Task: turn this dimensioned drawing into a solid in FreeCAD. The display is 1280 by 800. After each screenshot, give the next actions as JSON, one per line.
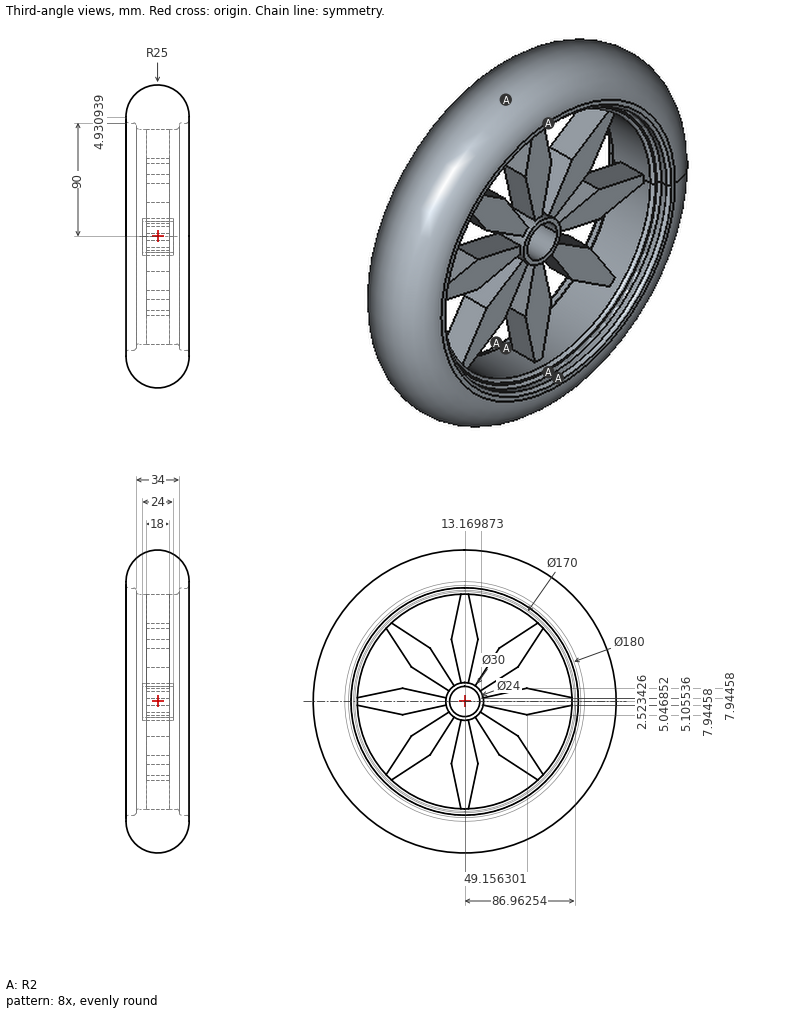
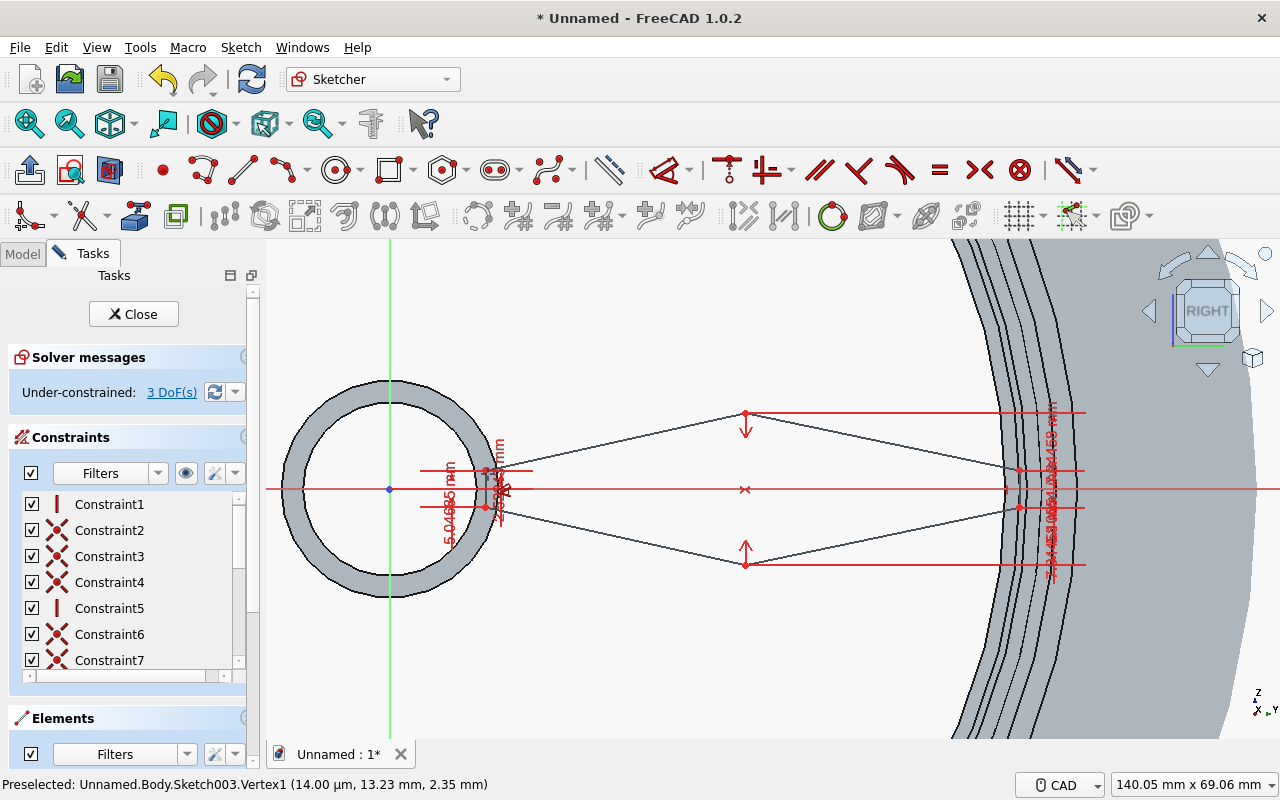
{"action": "left_click", "coordinate": [1020, 508]}
{"action": "left_click", "coordinate": [705, 542]}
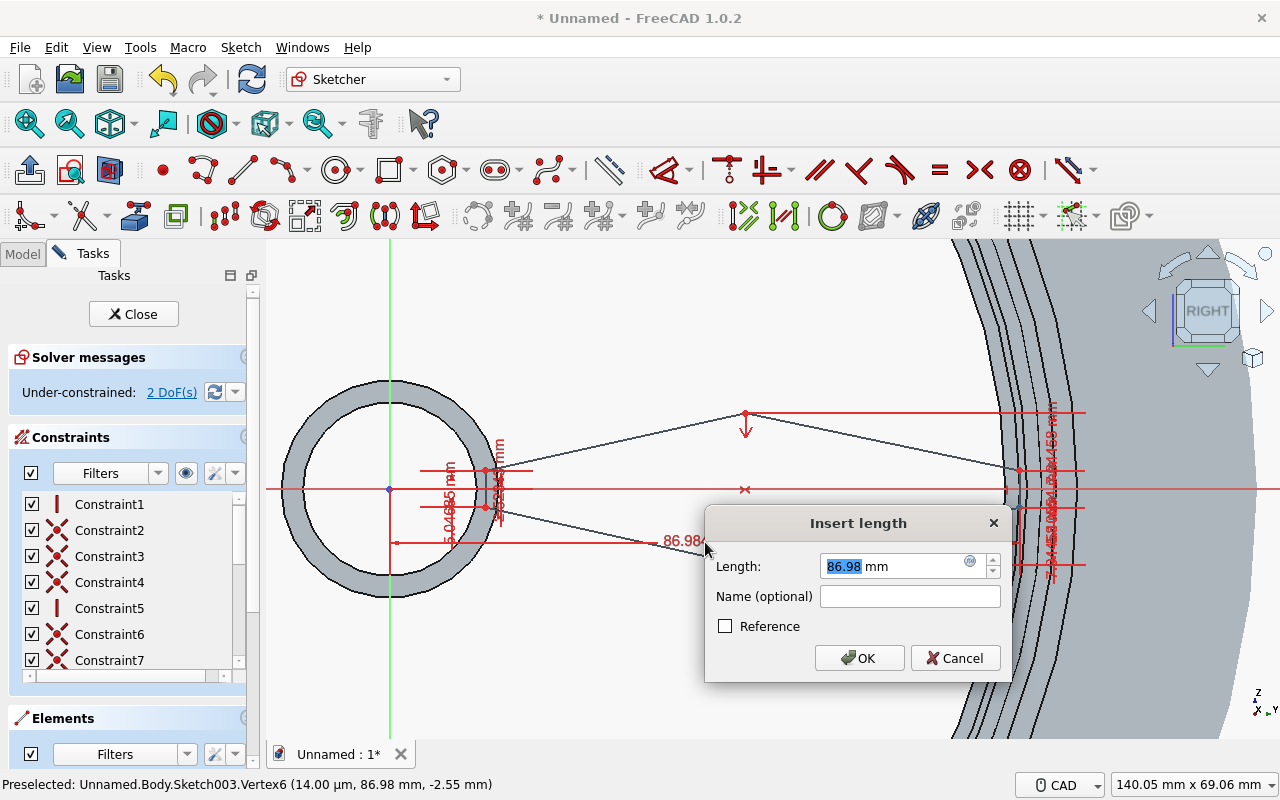
{"action": "type", "text": "86.96254"}
{"action": "key", "text": "Return"}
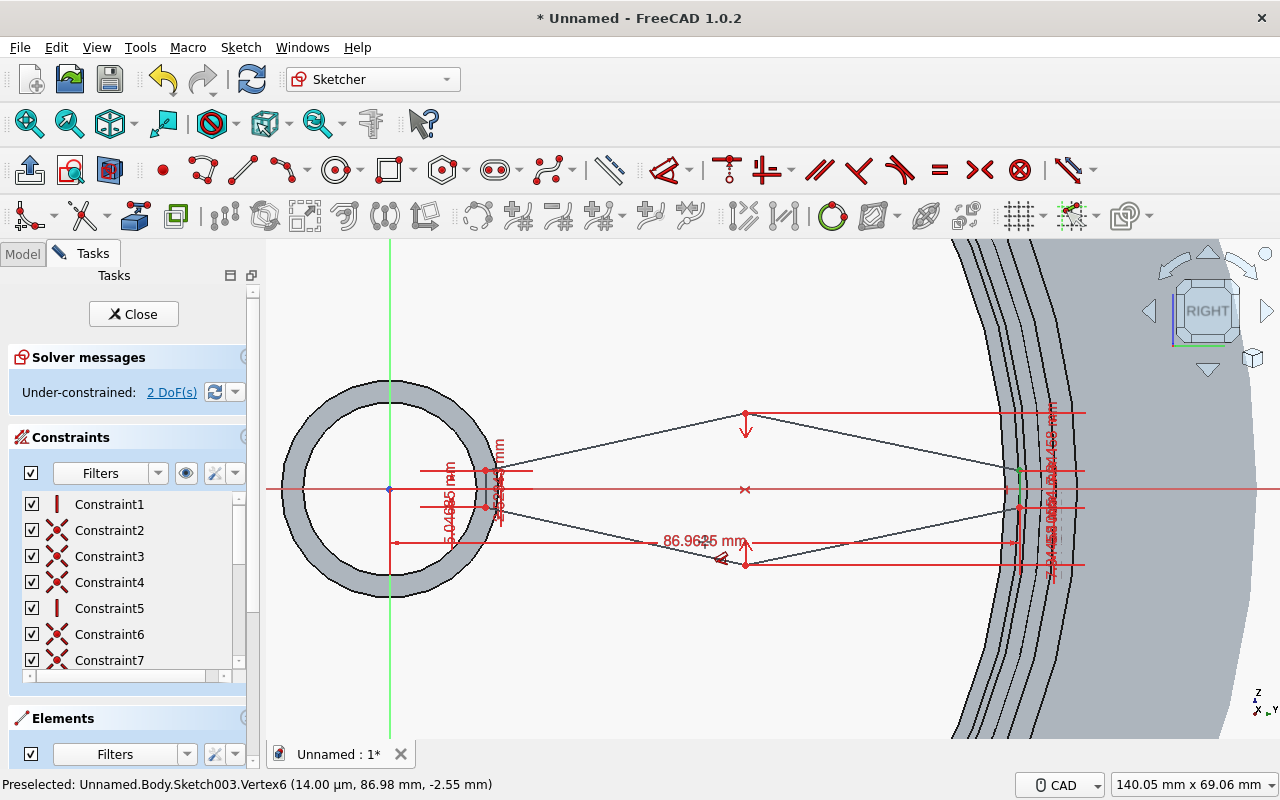
{"action": "left_click", "coordinate": [486, 471]}
{"action": "left_click", "coordinate": [438, 437]}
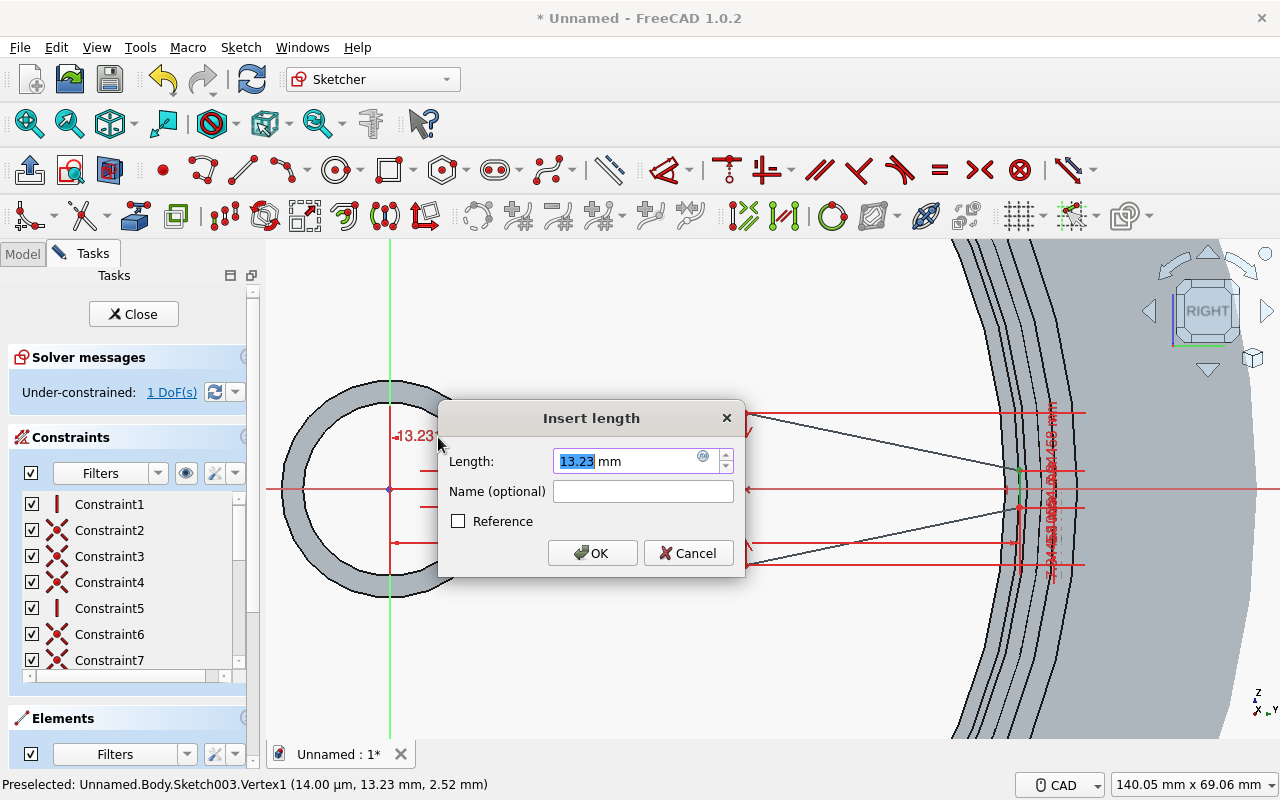
{"action": "type", "text": "13.169873"}
{"action": "key", "text": "Return"}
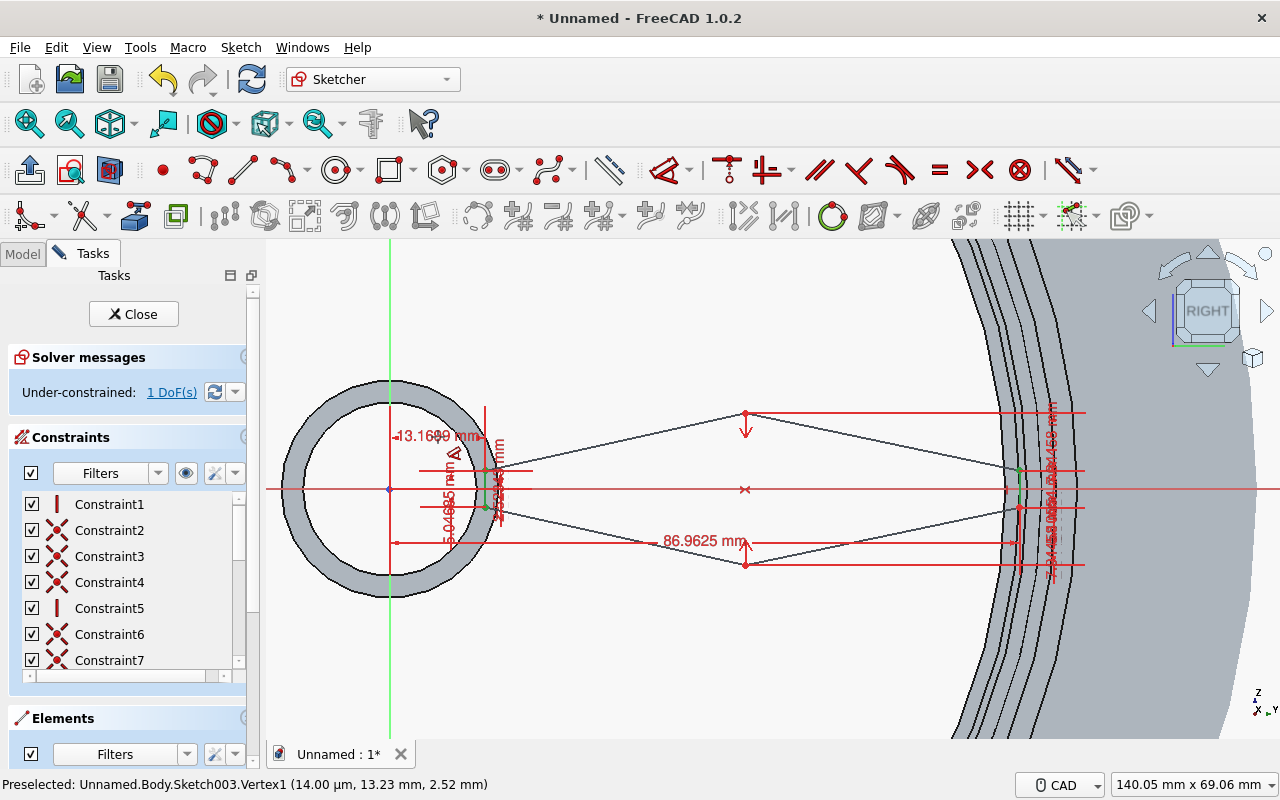
{"action": "left_click", "coordinate": [746, 565]}
{"action": "left_click", "coordinate": [568, 599]}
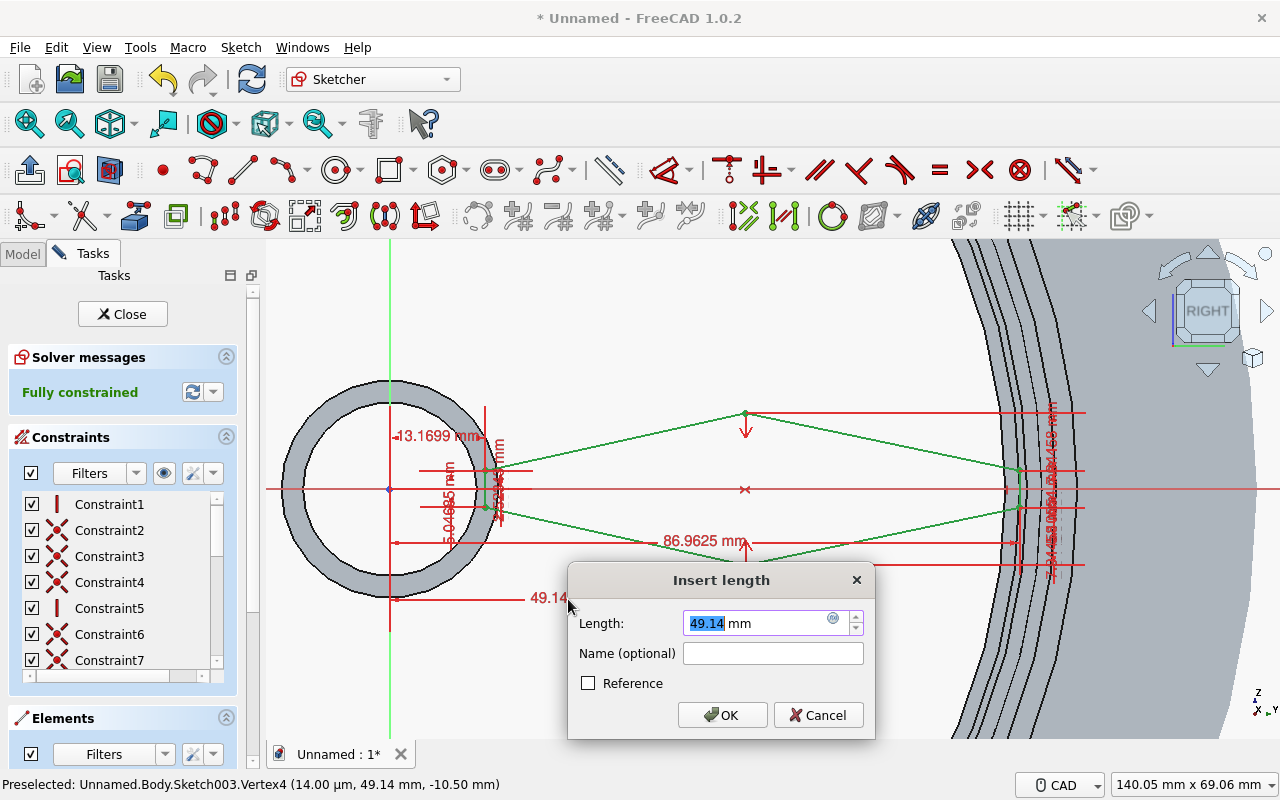
{"action": "type", "text": "49.156301"}
{"action": "key", "text": "Return"}
{"action": "key", "text": "Escape"}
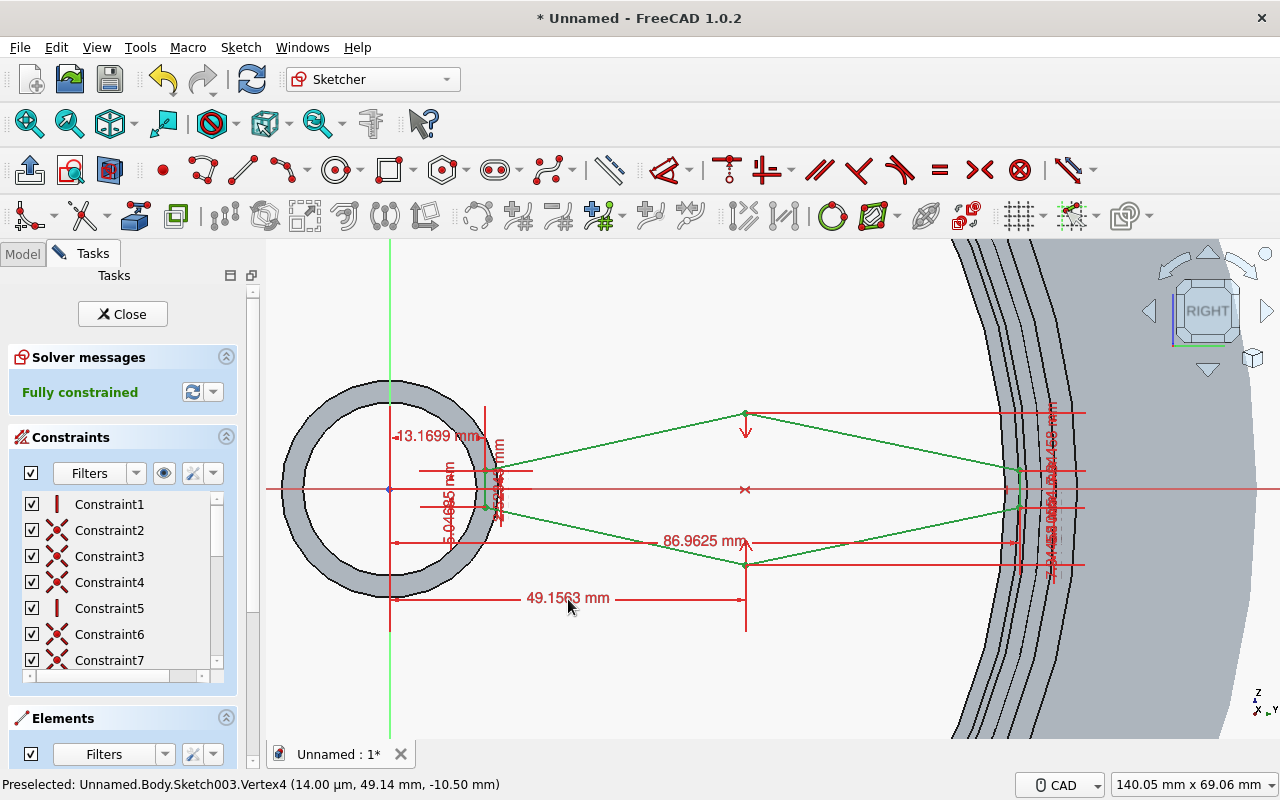
{"action": "left_click", "coordinate": [123, 314]}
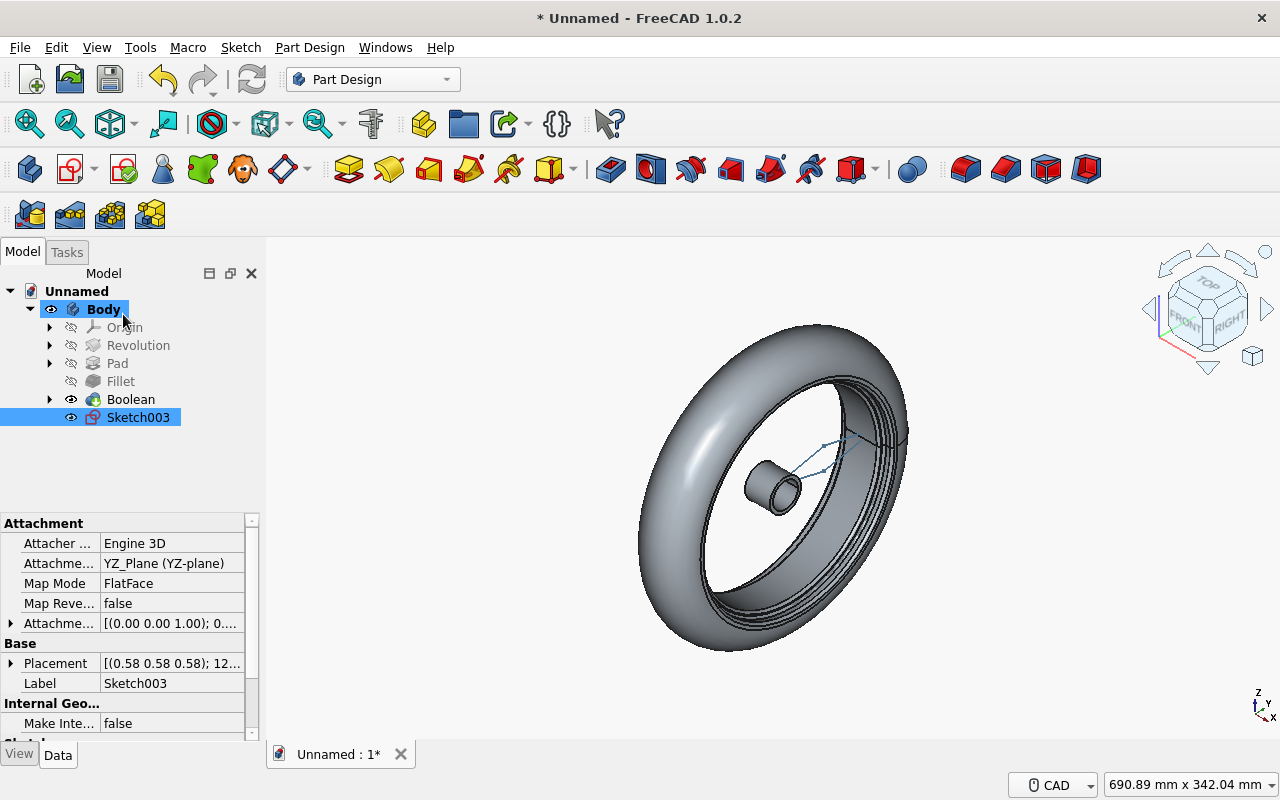
{"action": "left_click", "coordinate": [350, 170]}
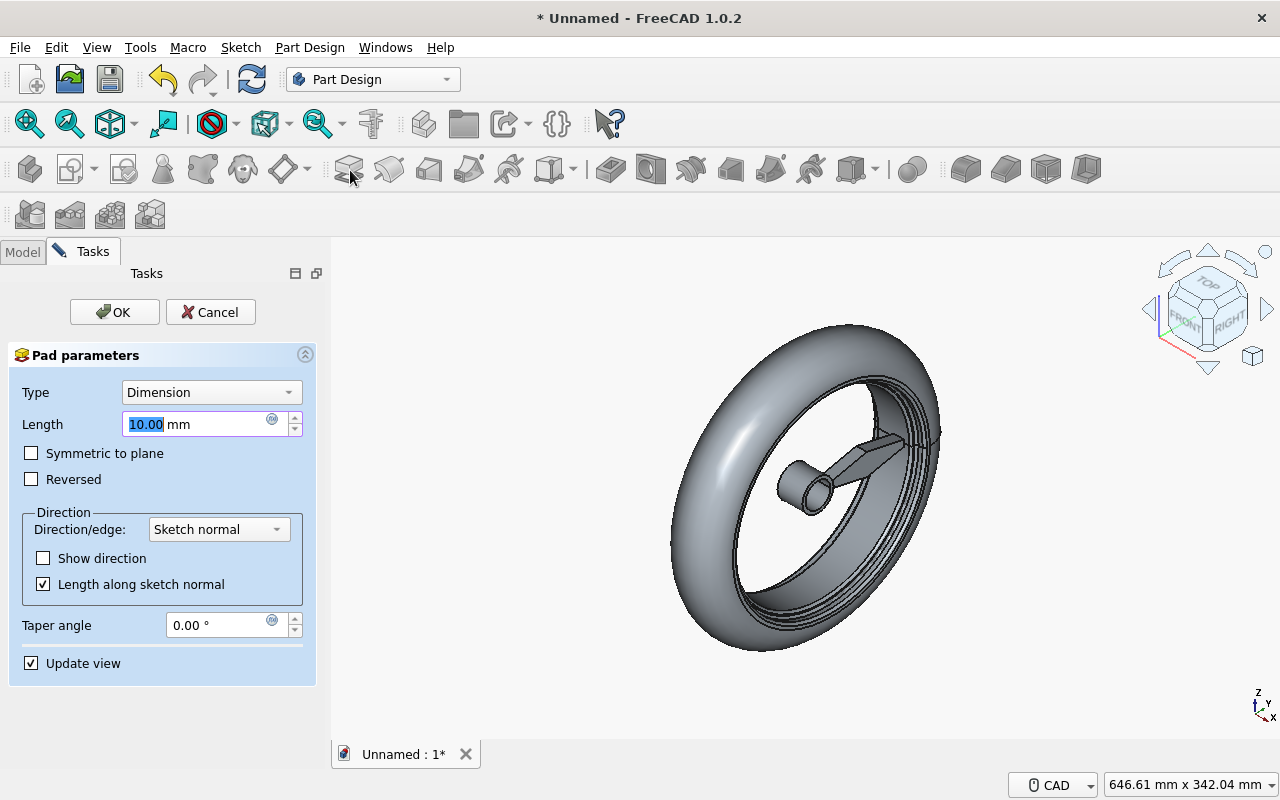
{"action": "type", "text": "18"}
{"action": "key", "text": "Tab"}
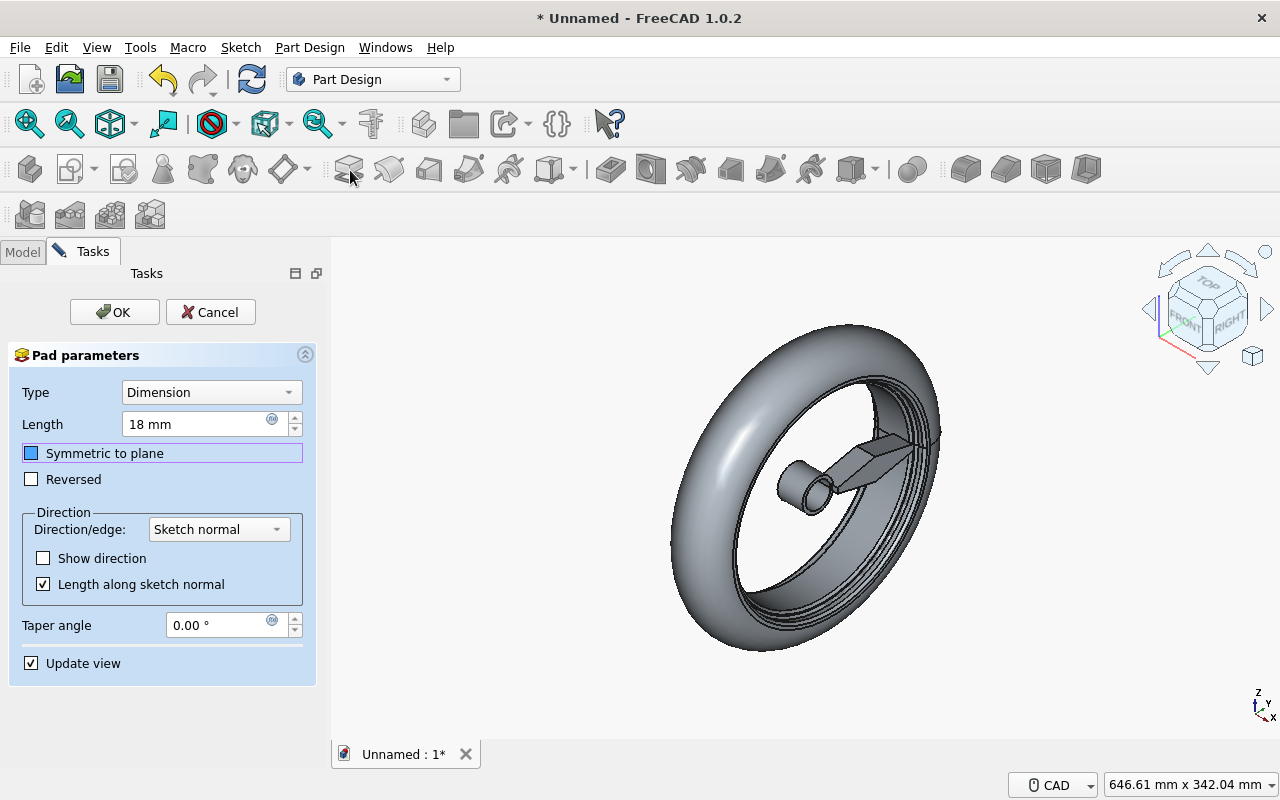
{"action": "left_click", "coordinate": [30, 453]}